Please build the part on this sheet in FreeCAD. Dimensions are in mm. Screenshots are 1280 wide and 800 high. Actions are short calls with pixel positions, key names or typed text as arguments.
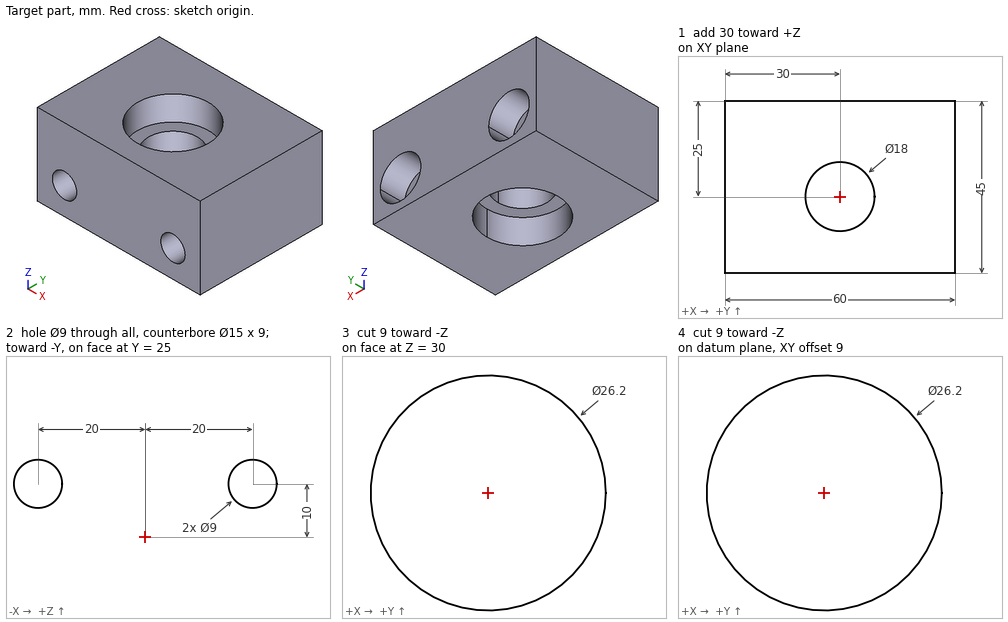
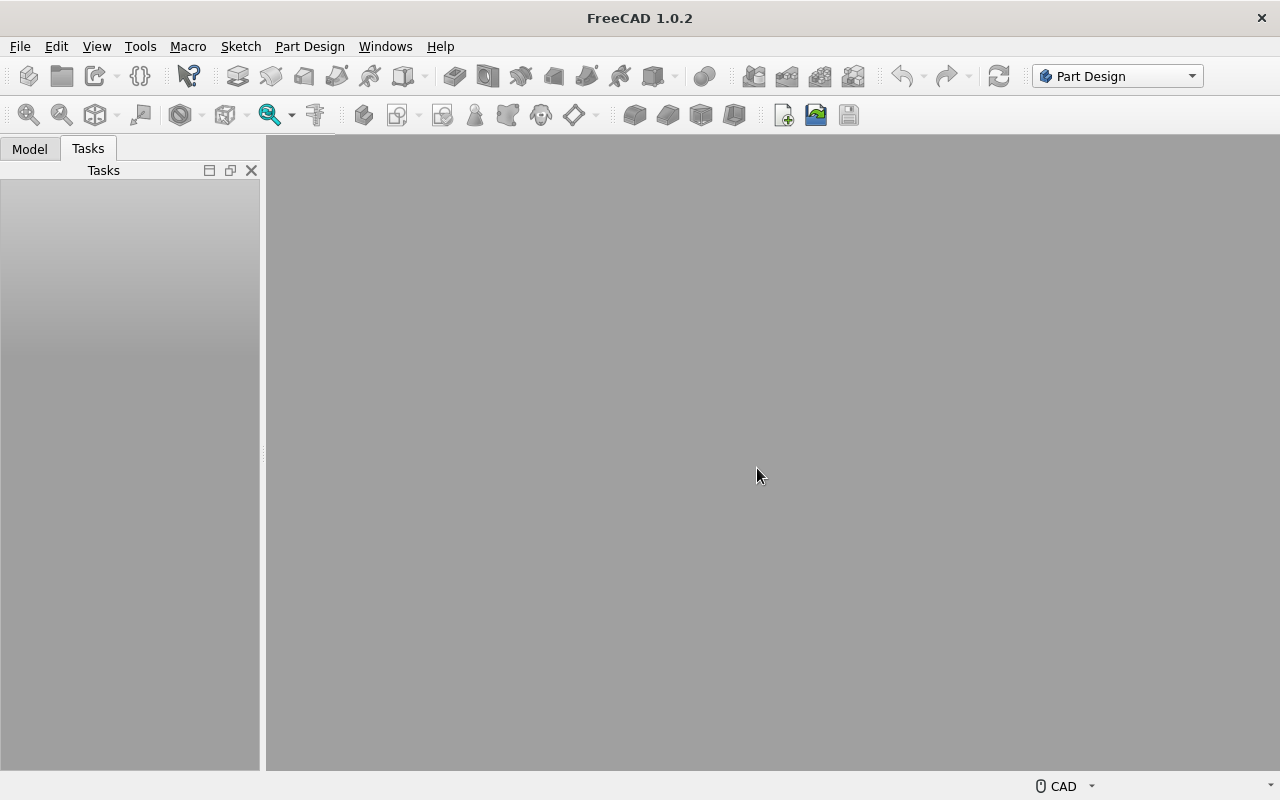
click(783, 116)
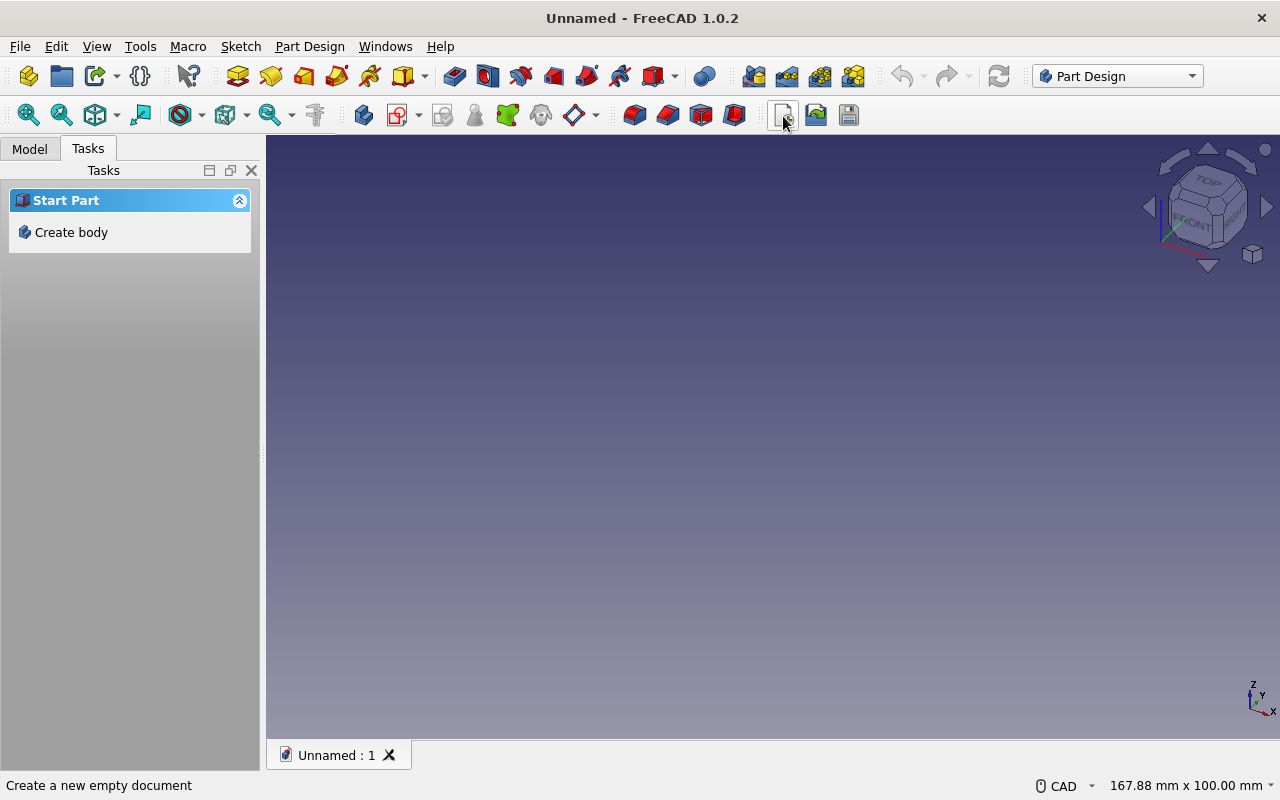
click(396, 116)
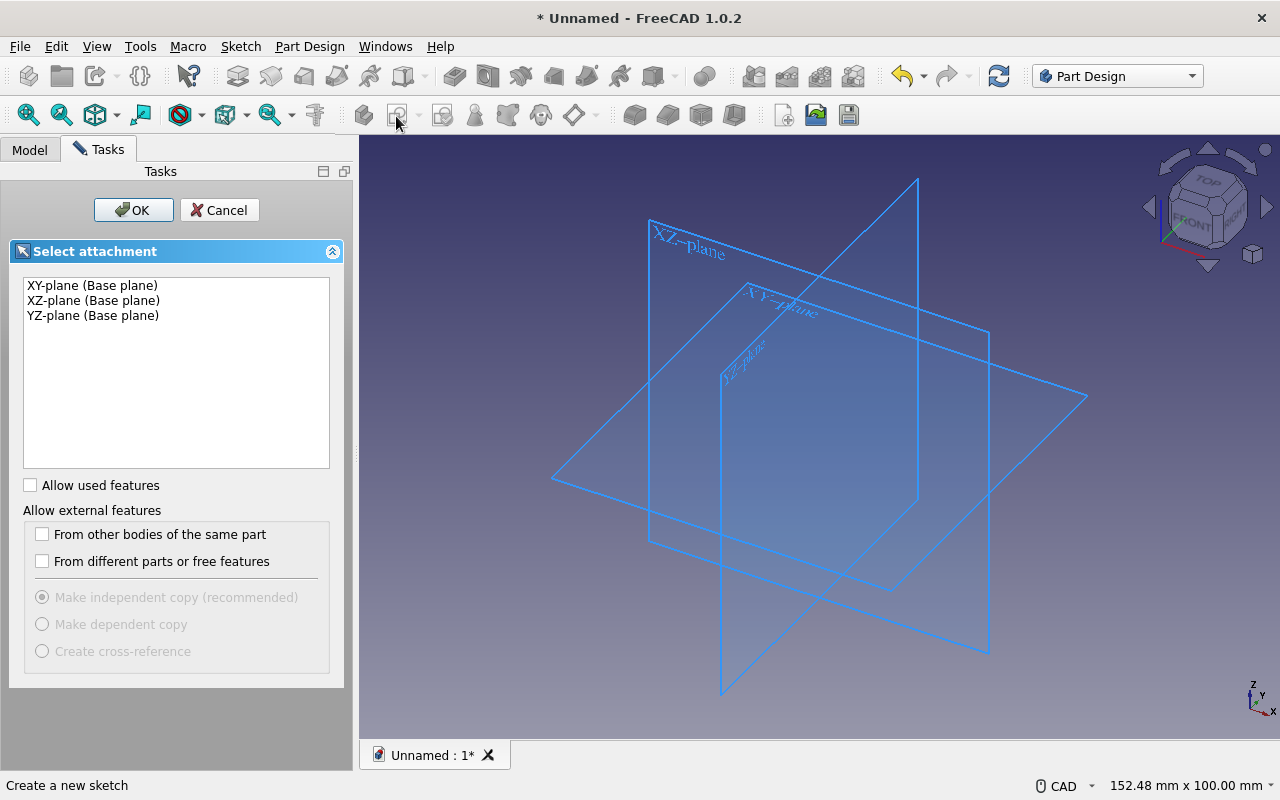
click(84, 286)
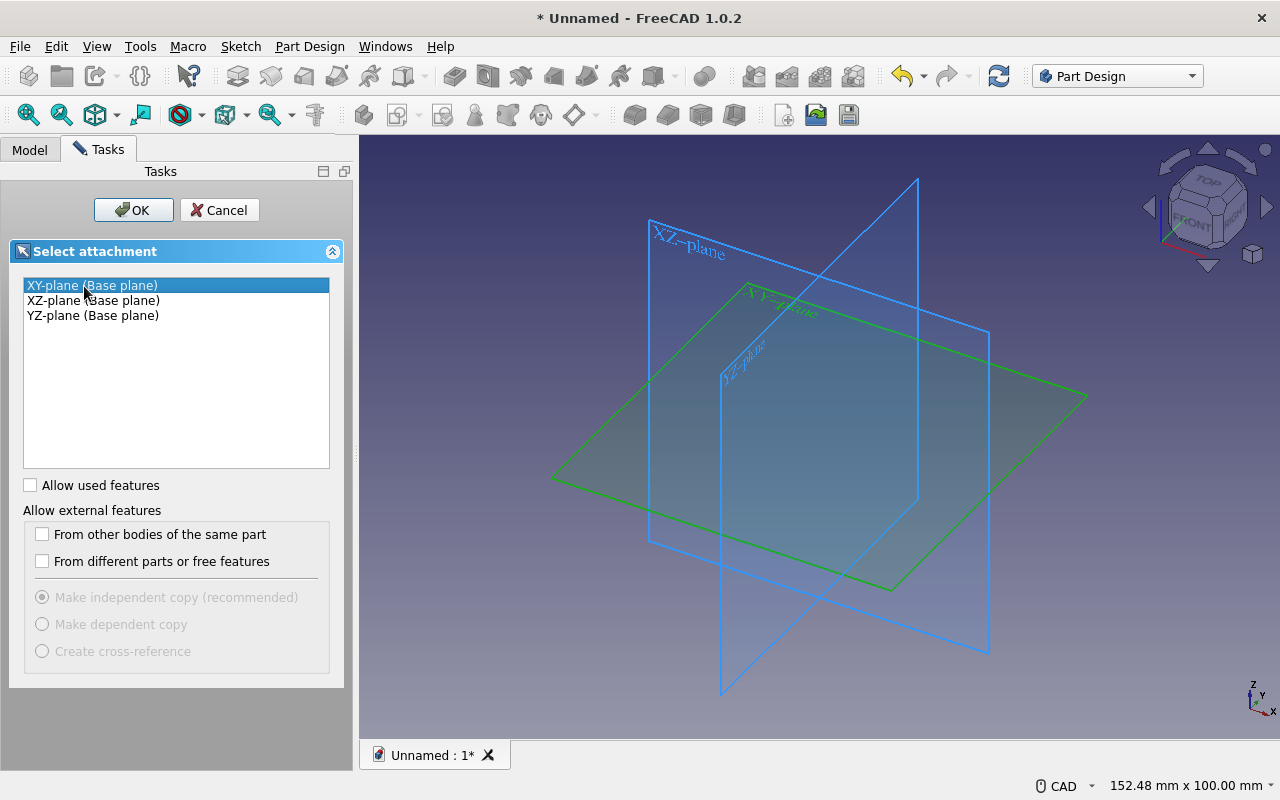
click(134, 210)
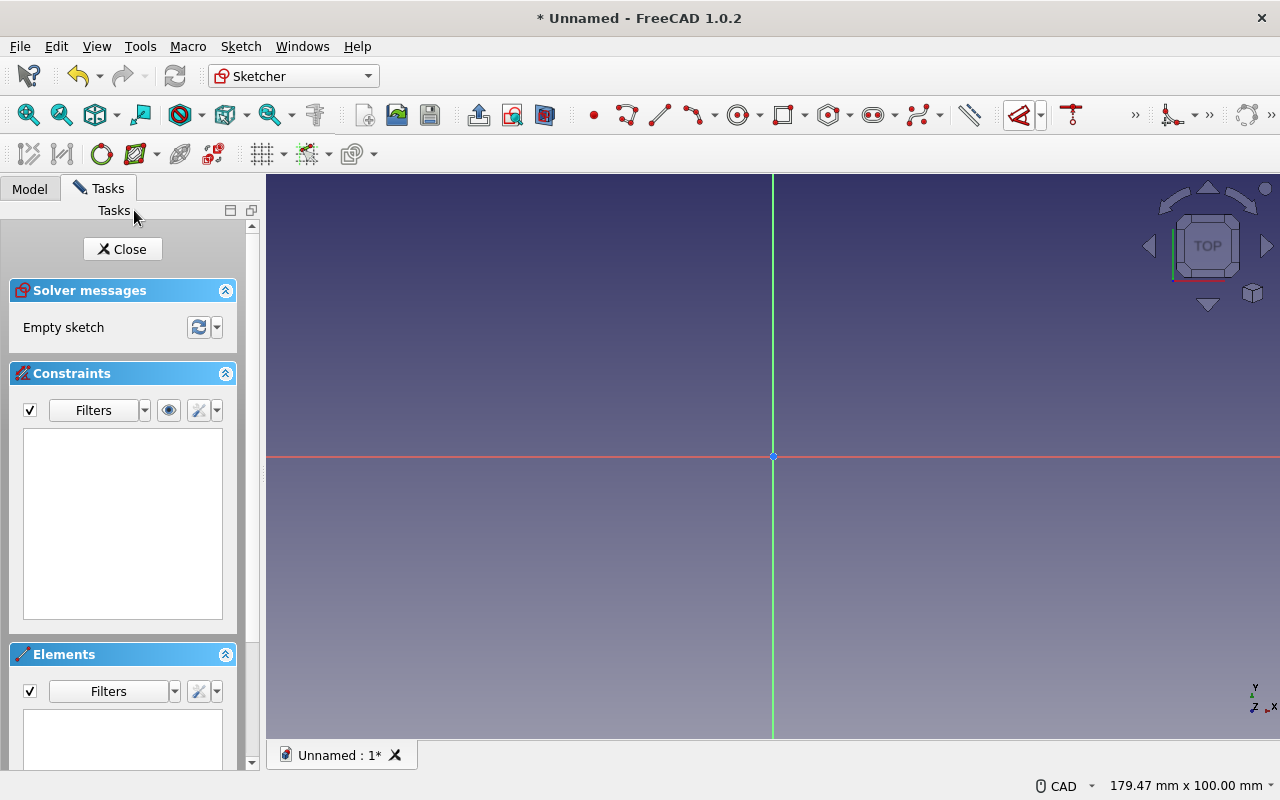
scroll(912, 414, up, 2)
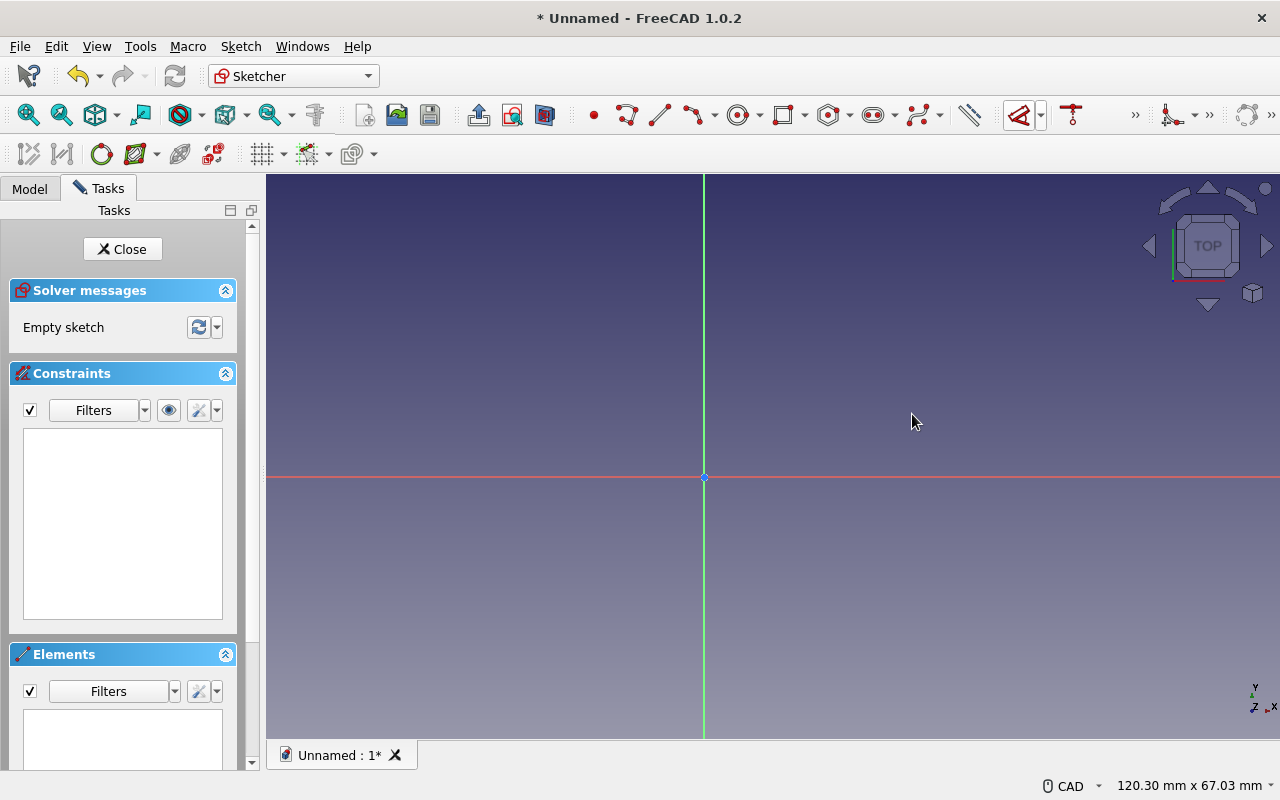
click(782, 116)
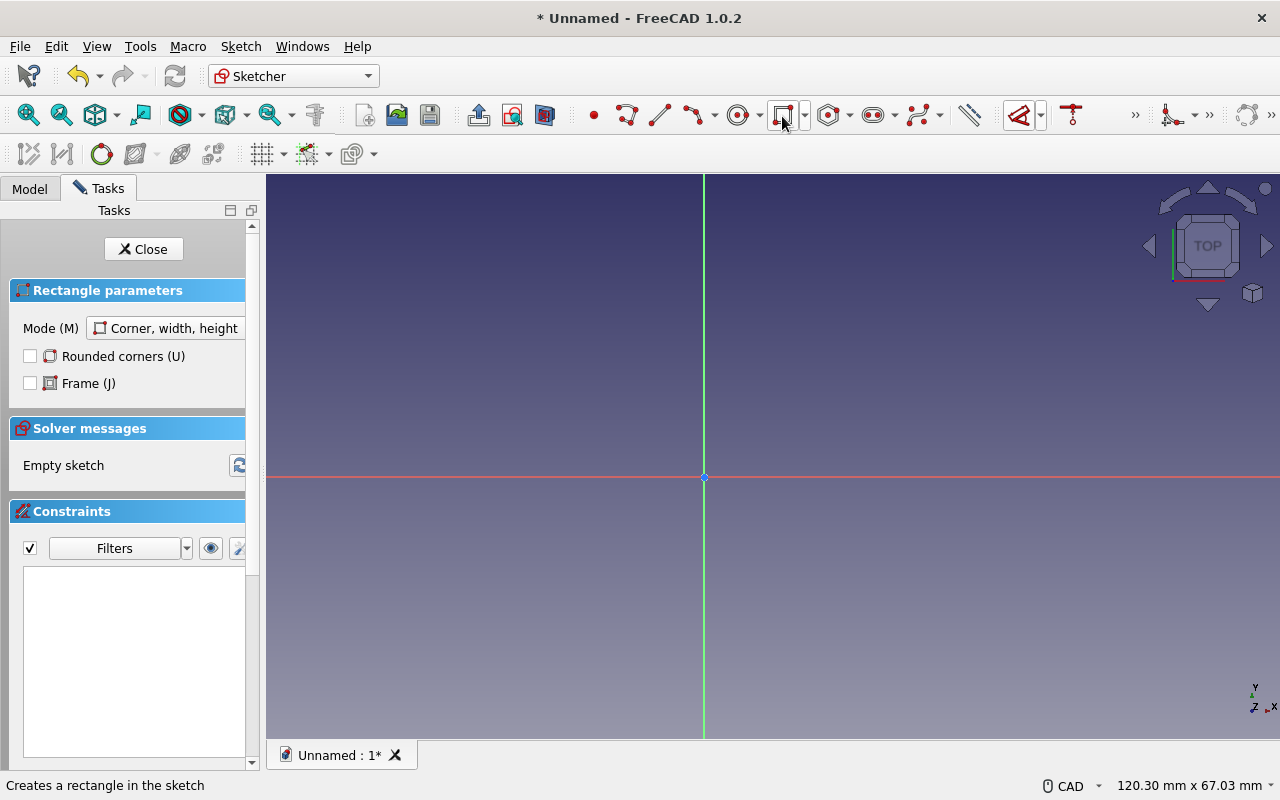
click(451, 266)
move(957, 646)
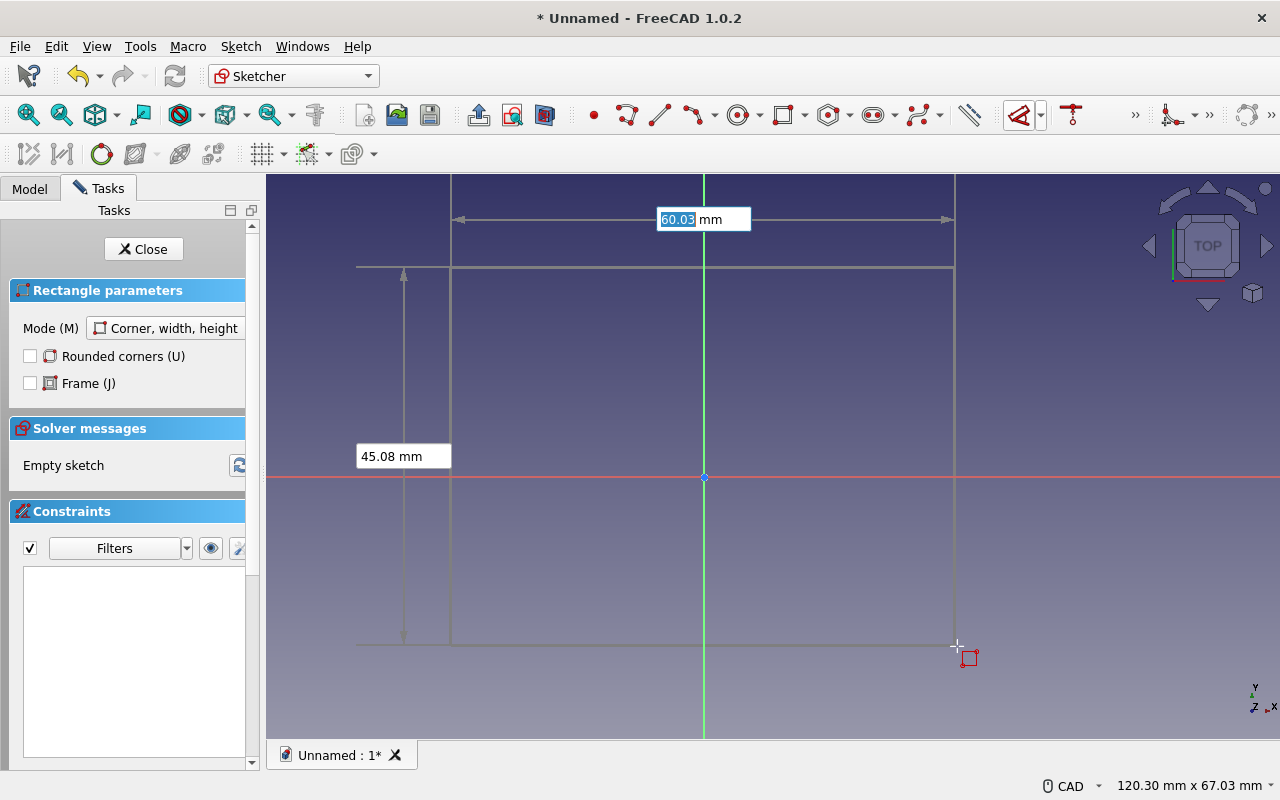
text(60)
key(Tab)
text(45)
key(Return)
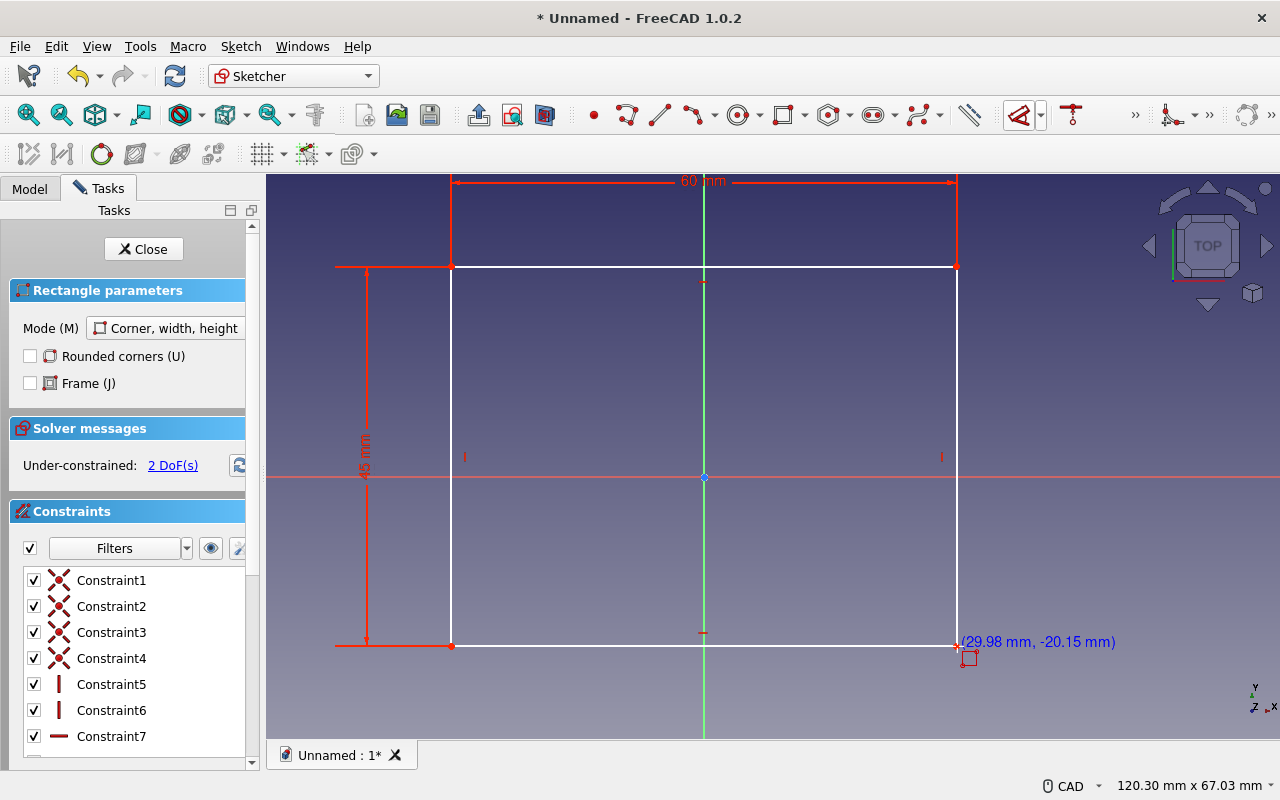
click(738, 116)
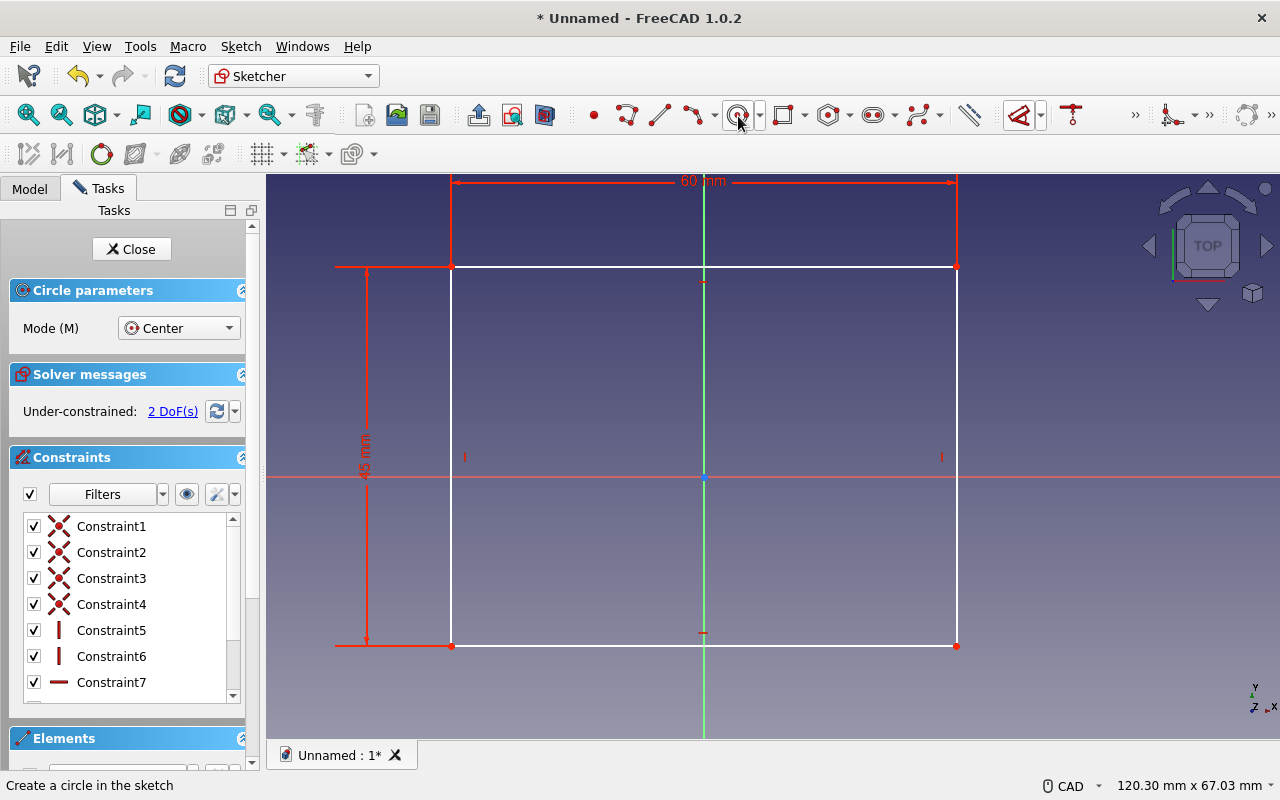
click(704, 477)
move(758, 424)